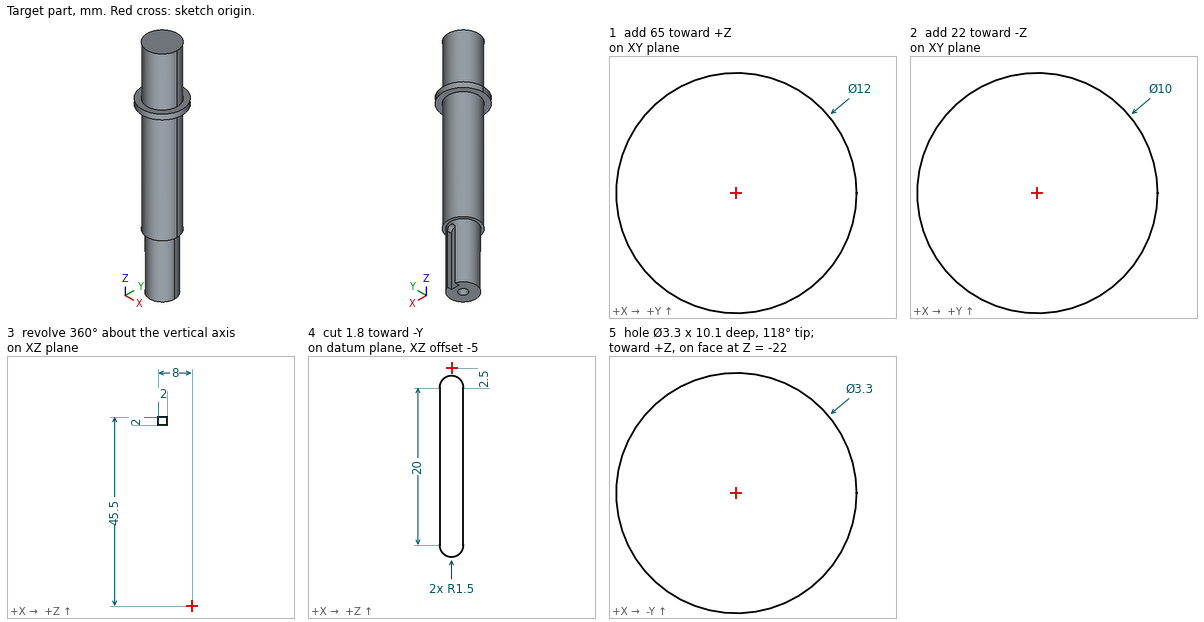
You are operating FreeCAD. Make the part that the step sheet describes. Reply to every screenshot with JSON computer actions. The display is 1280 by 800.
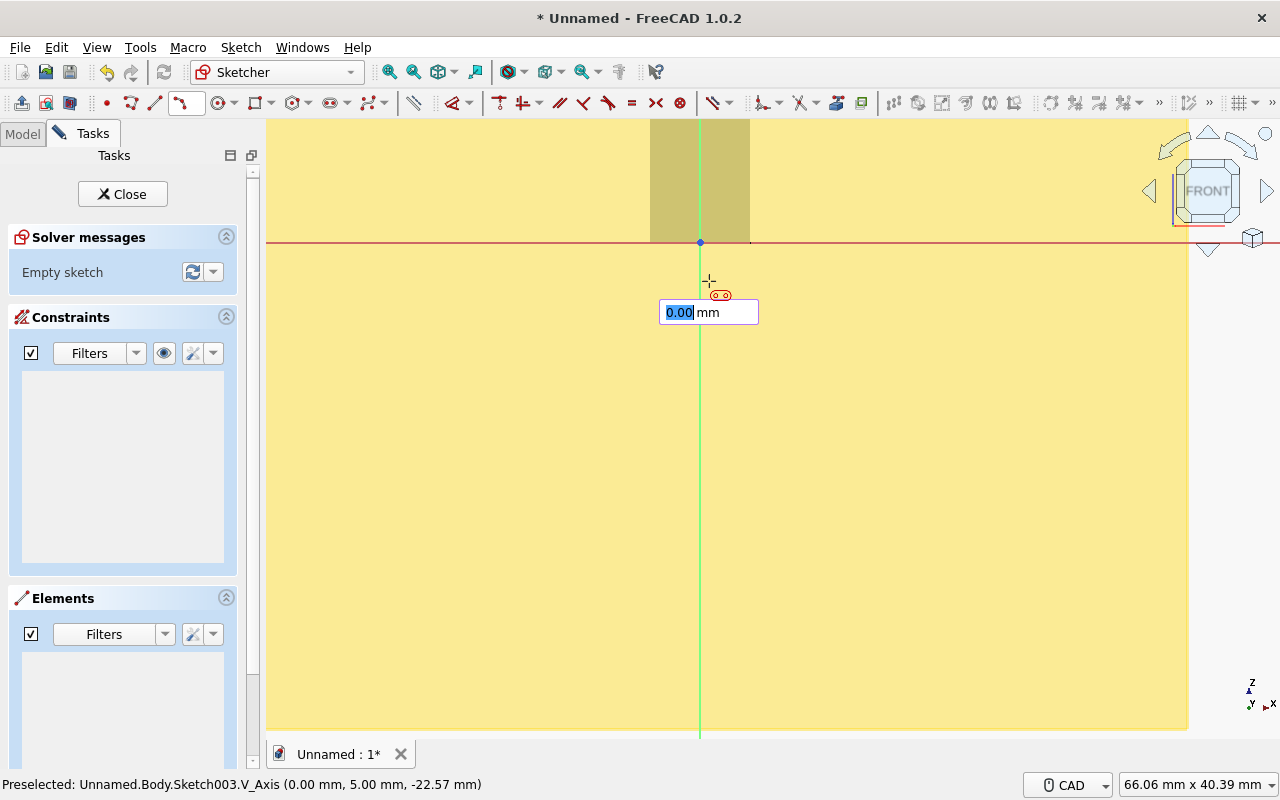
{"action": "left_click", "coordinate": [723, 434]}
{"action": "key", "text": "Escape"}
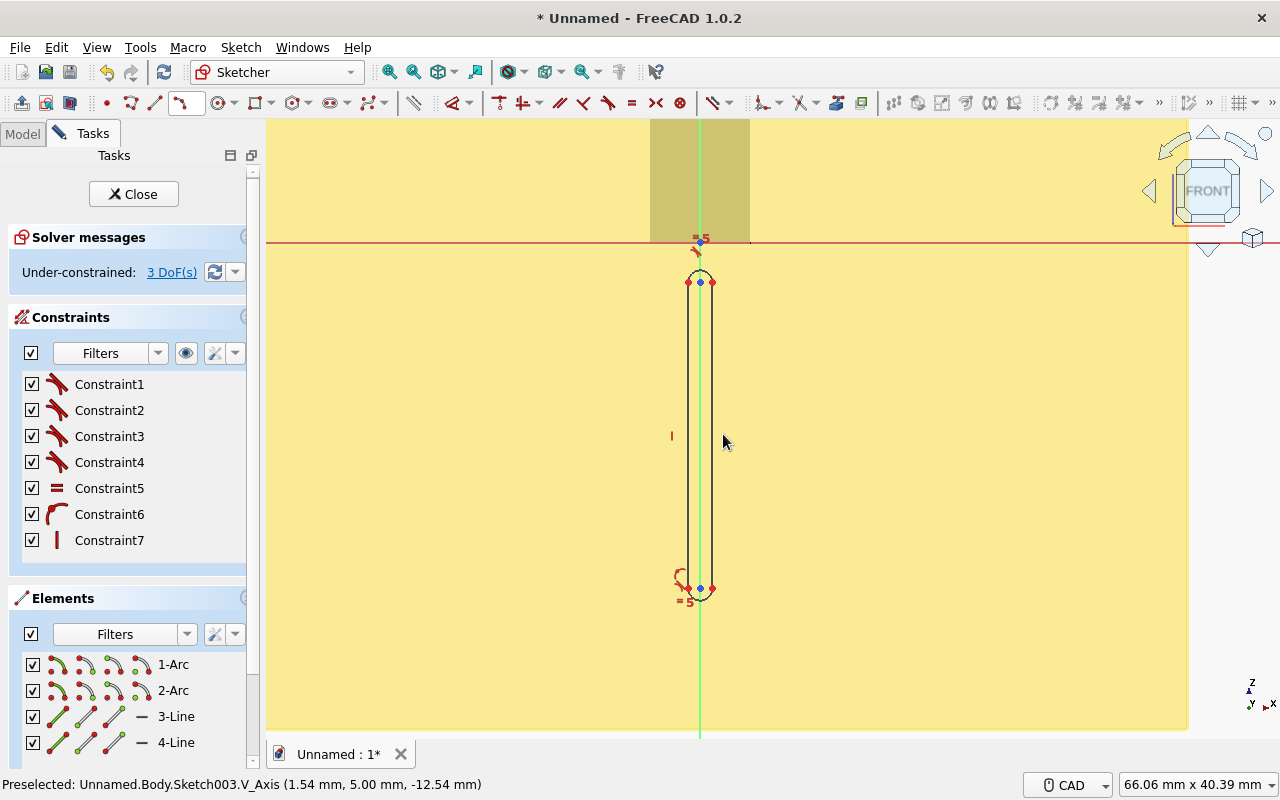
{"action": "left_click", "coordinate": [452, 104]}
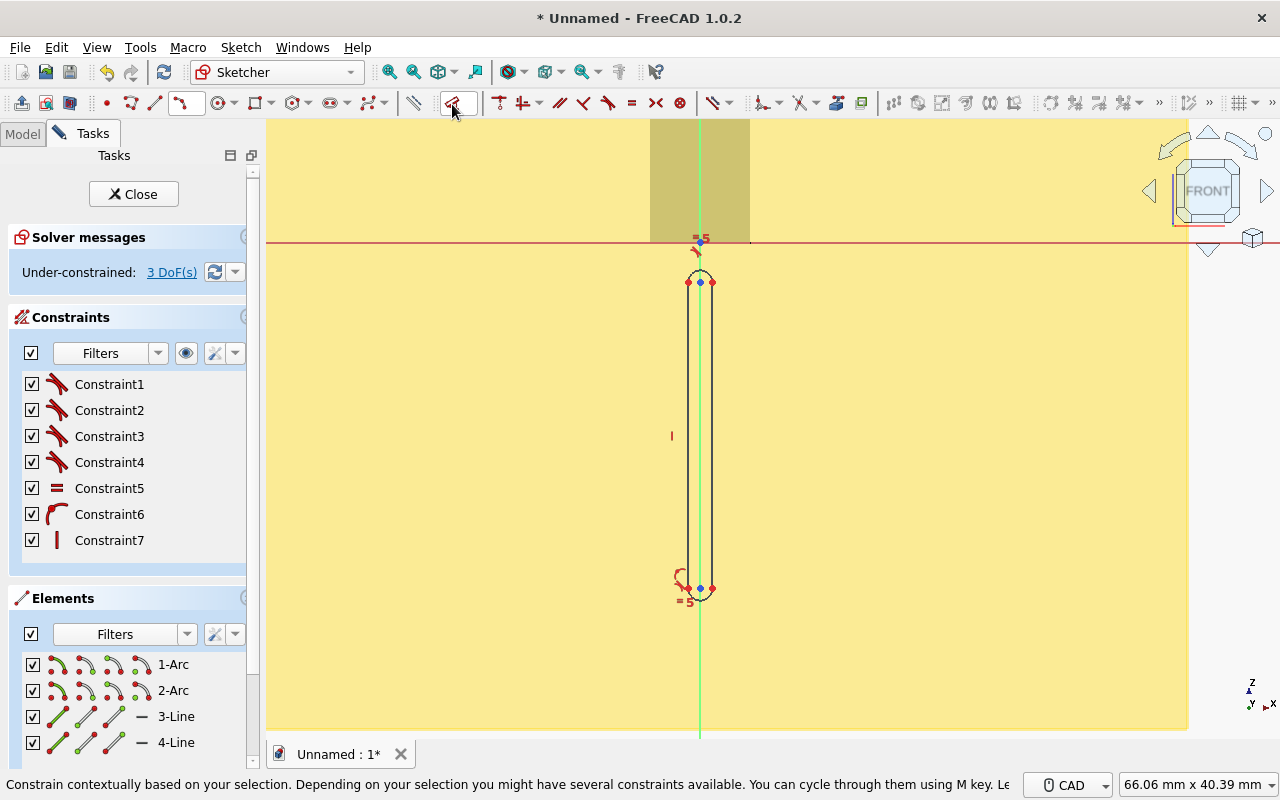
{"action": "scroll", "coordinate": [700, 601], "scroll_direction": "up", "scroll_amount": 3}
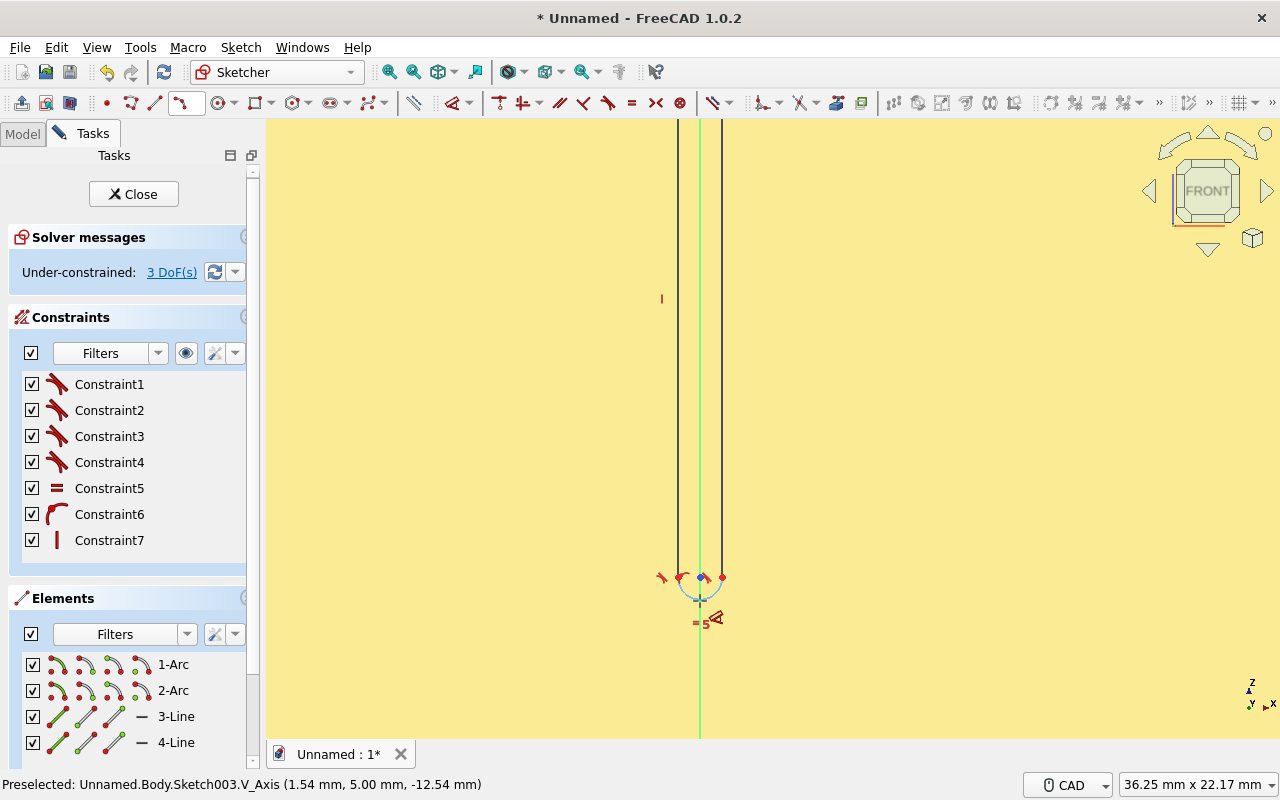
{"action": "left_click", "coordinate": [700, 600]}
{"action": "left_click", "coordinate": [674, 625]}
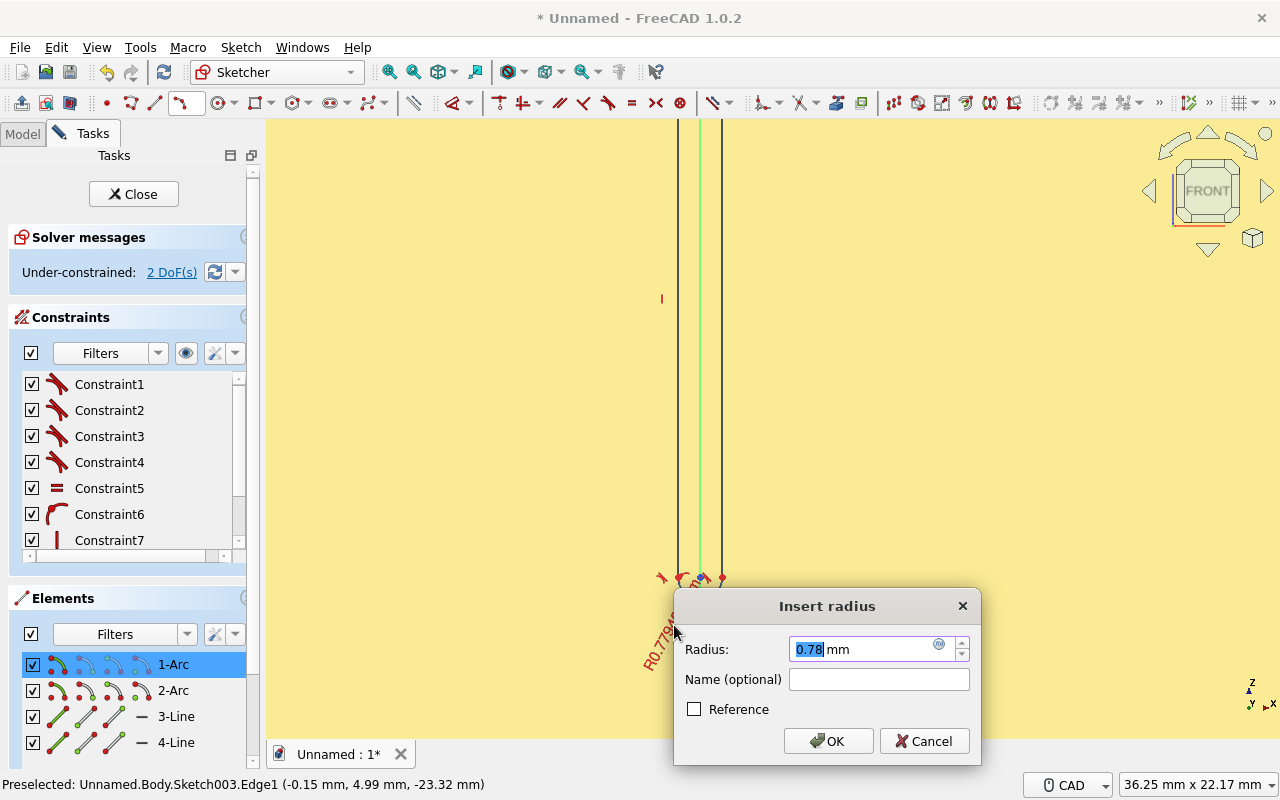
{"action": "type", "text": "1.5"}
{"action": "key", "text": "Return"}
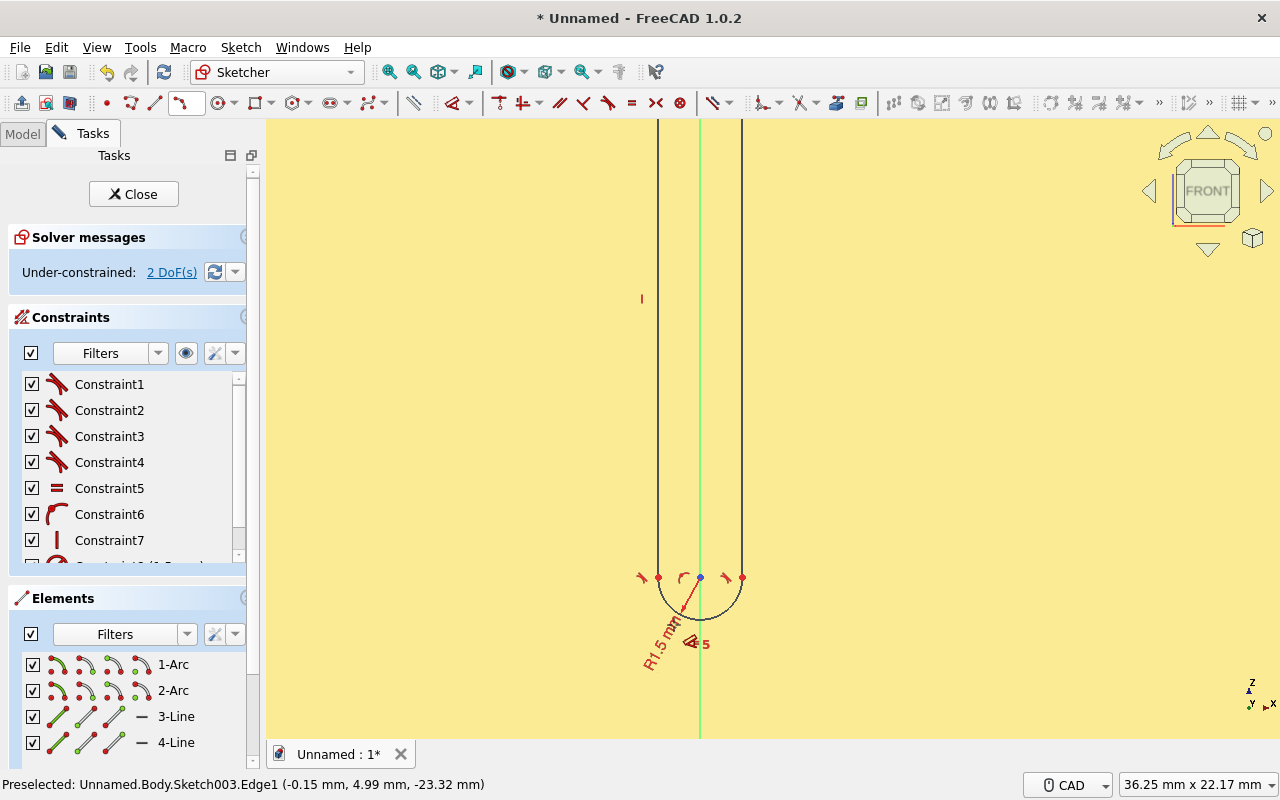
{"action": "left_click", "coordinate": [658, 410]}
{"action": "left_click", "coordinate": [624, 362]}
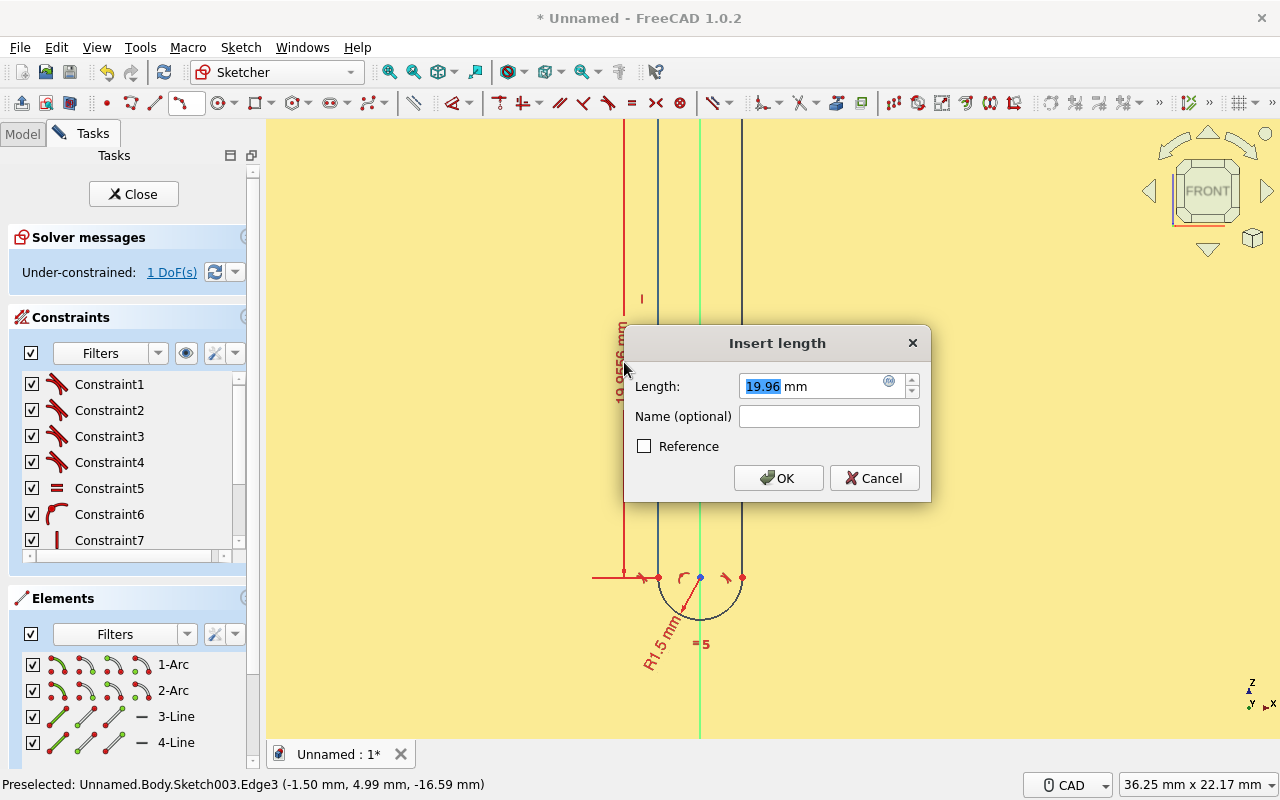
{"action": "type", "text": "20"}
{"action": "key", "text": "Return"}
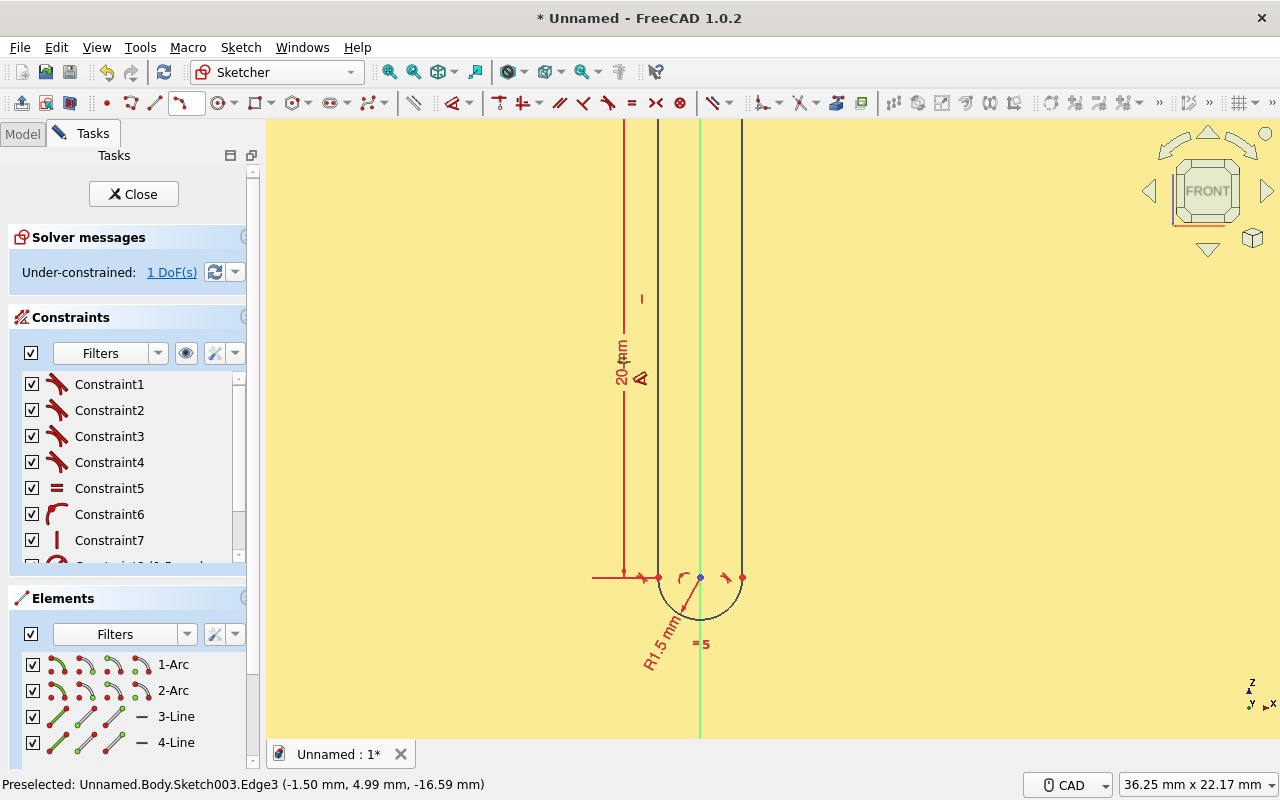
{"action": "scroll", "coordinate": [710, 607], "scroll_direction": "down", "scroll_amount": 3}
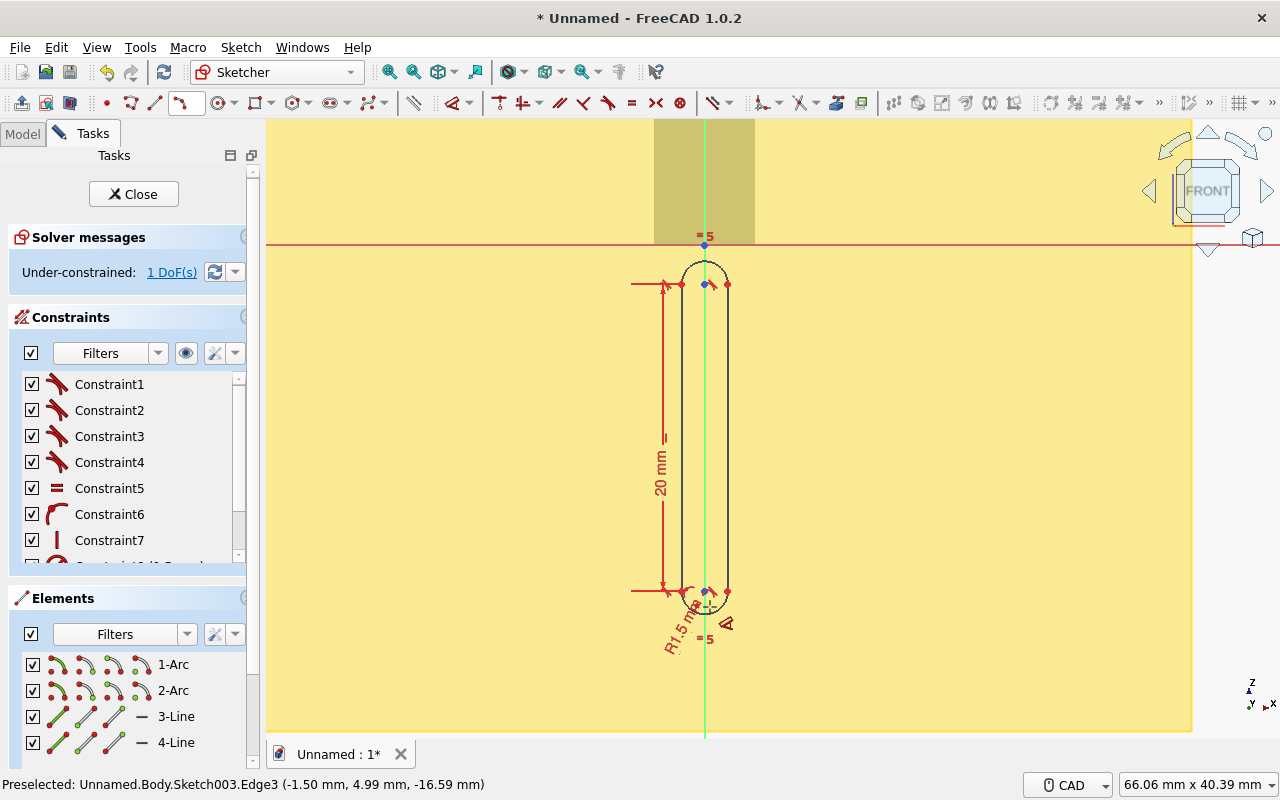
{"action": "left_click", "coordinate": [728, 284]}
{"action": "left_click", "coordinate": [762, 265]}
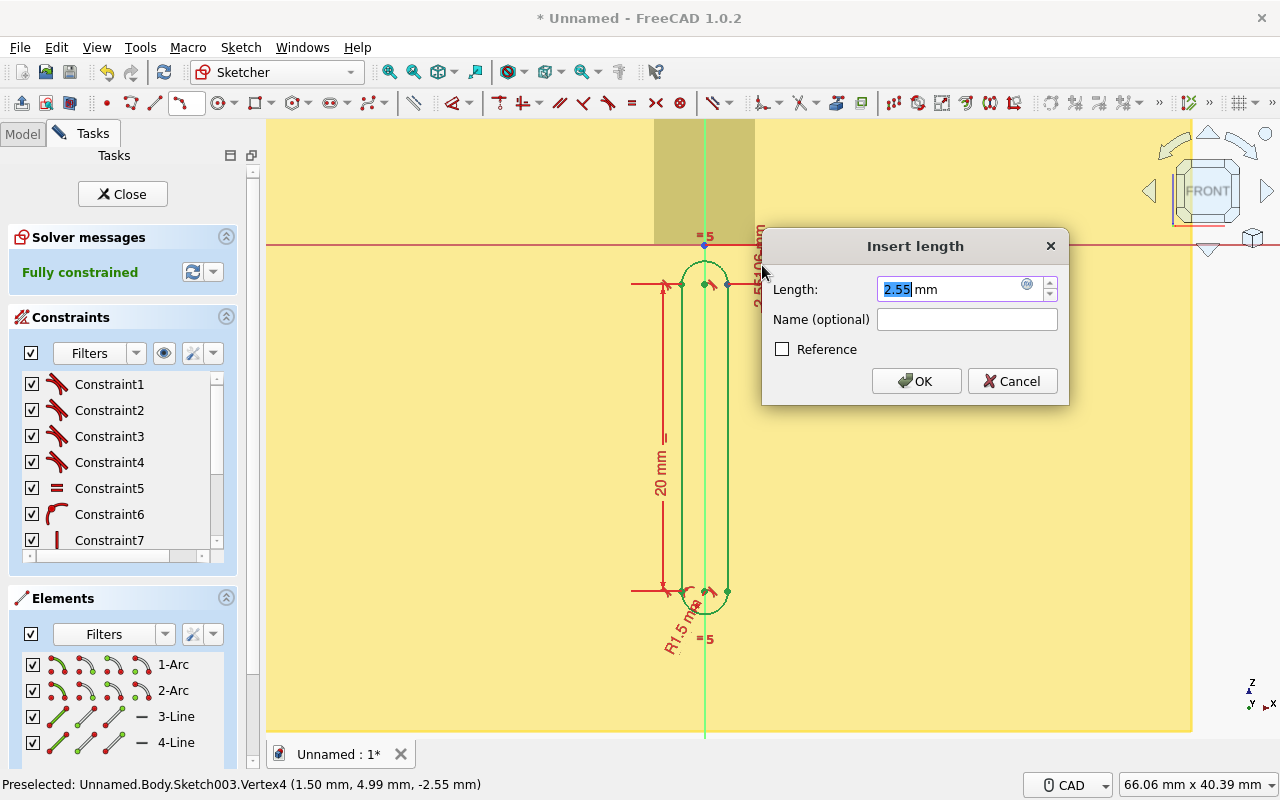
{"action": "type", "text": "2.5"}
{"action": "key", "text": "Return"}
{"action": "key", "text": "Escape"}